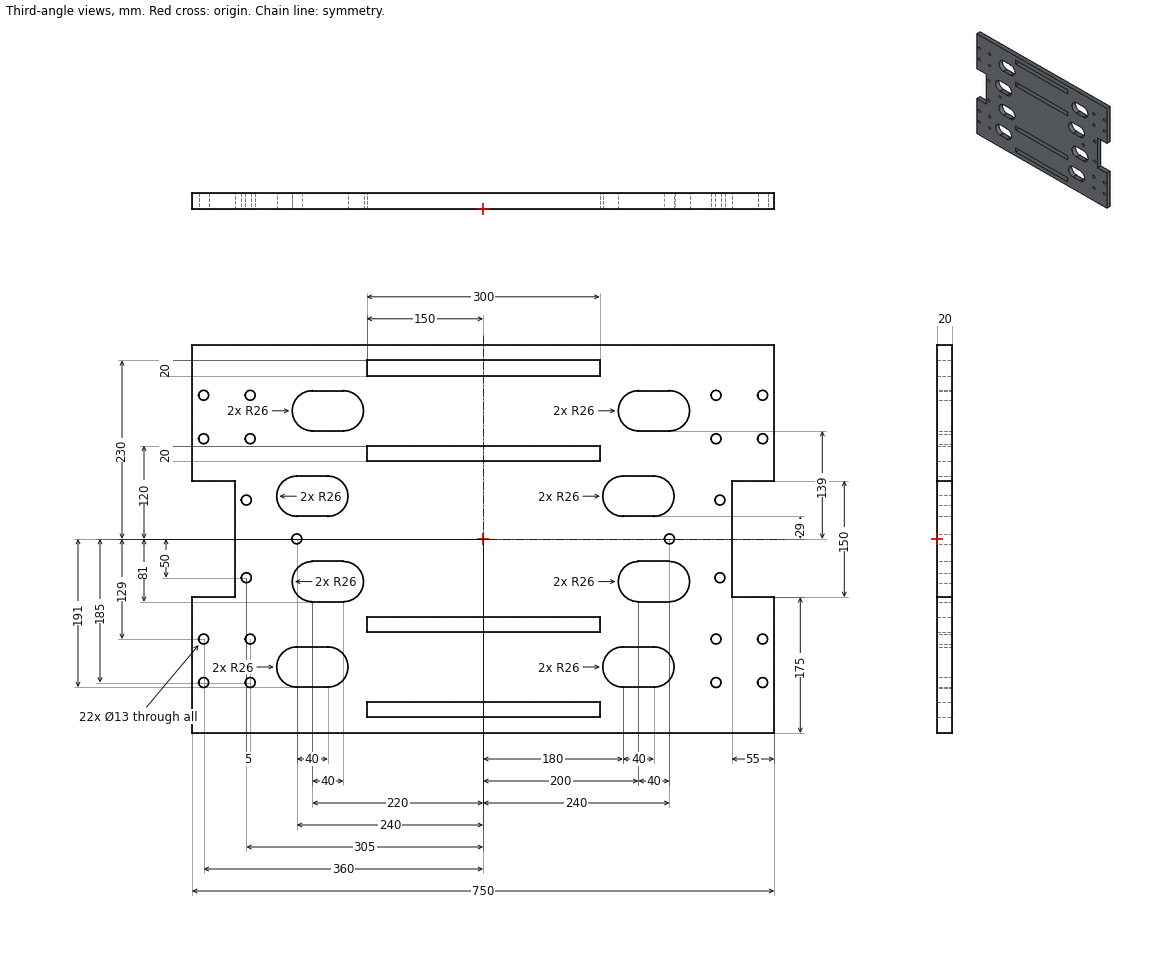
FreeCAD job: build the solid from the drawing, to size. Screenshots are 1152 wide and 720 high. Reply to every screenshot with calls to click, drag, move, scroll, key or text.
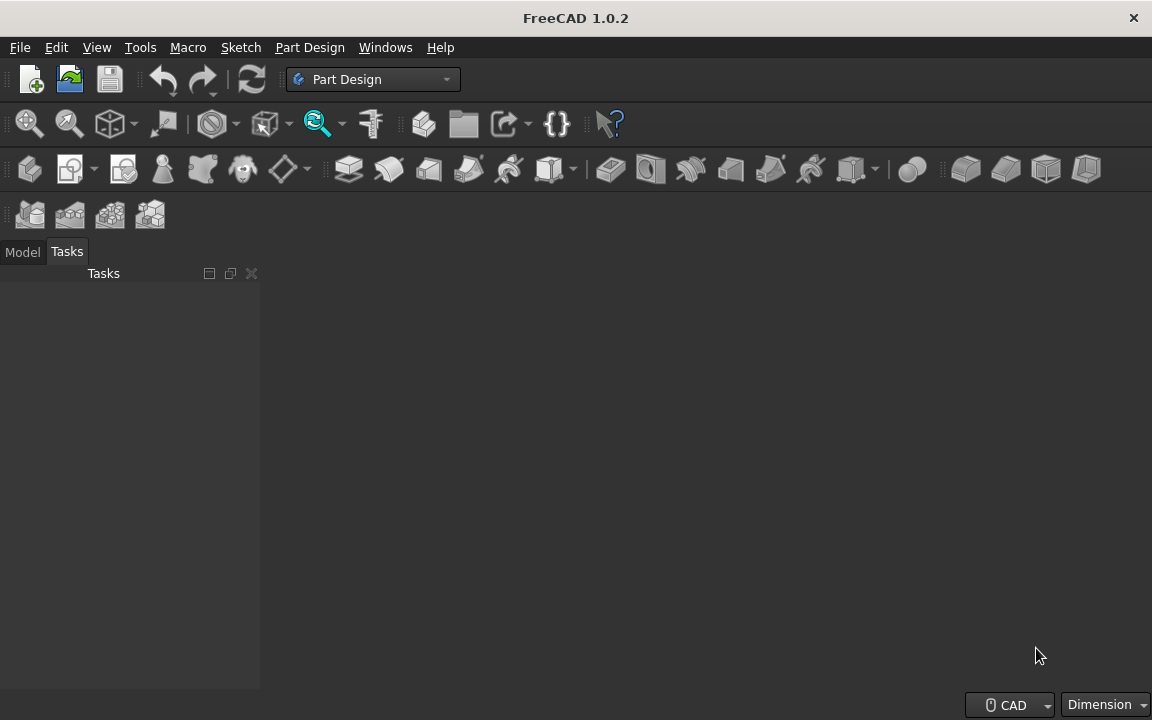
click(30, 80)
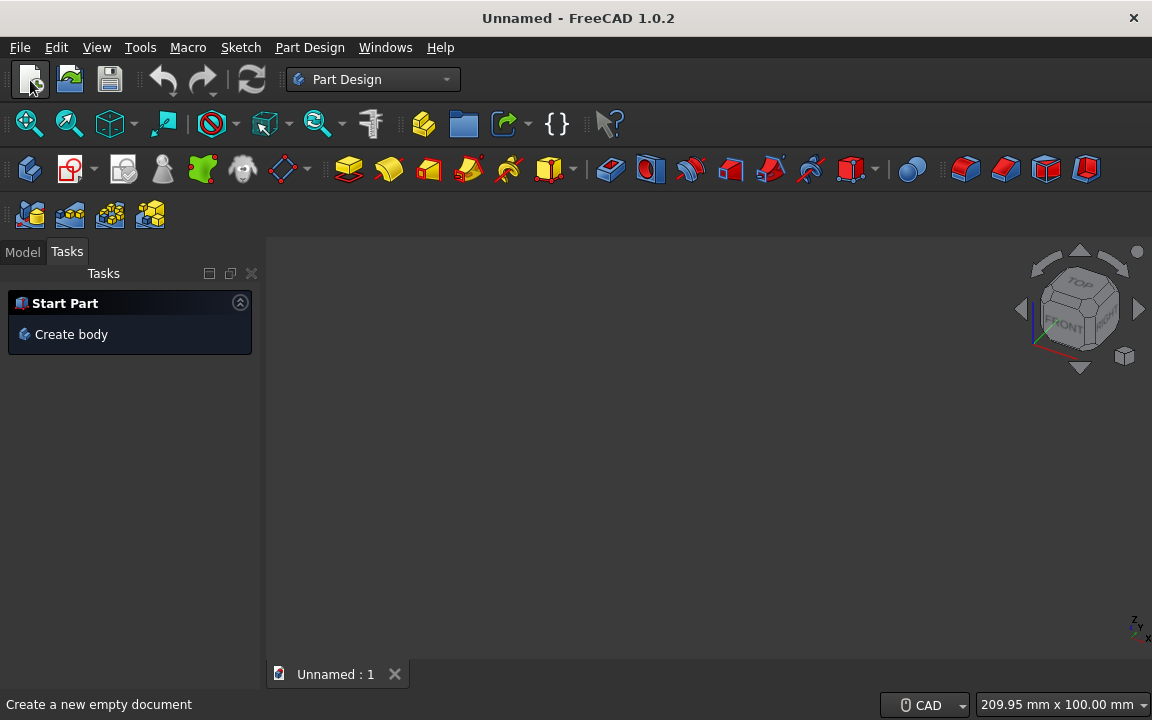
click(70, 170)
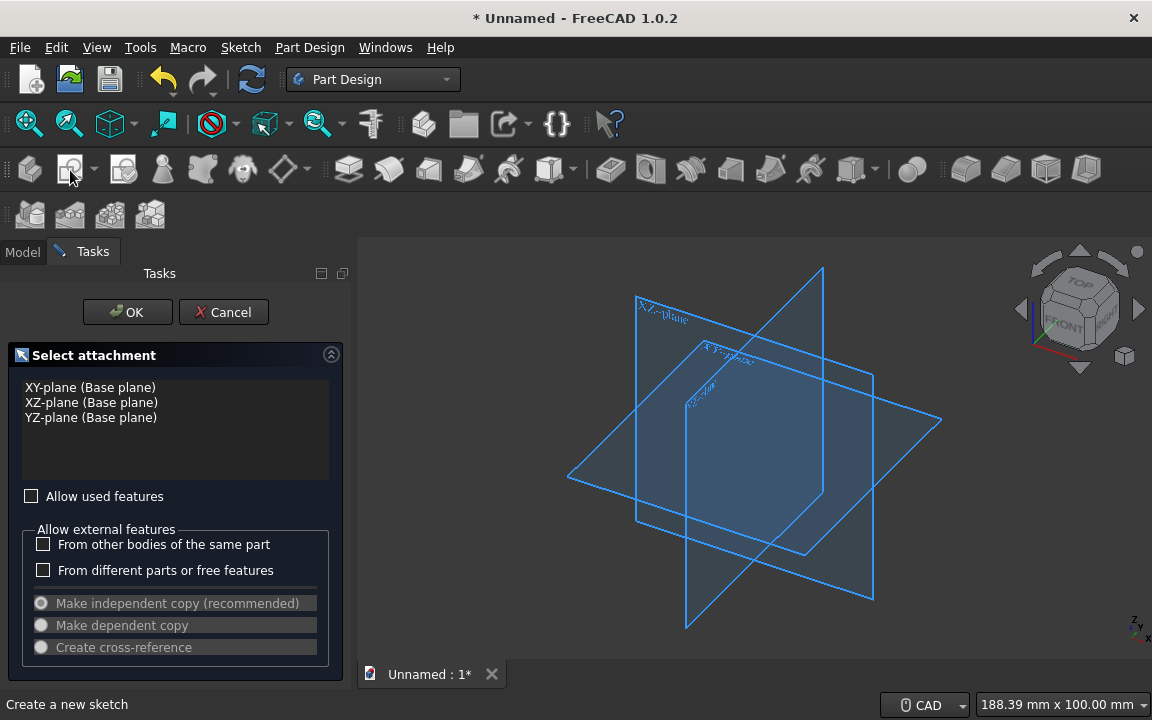
click(82, 402)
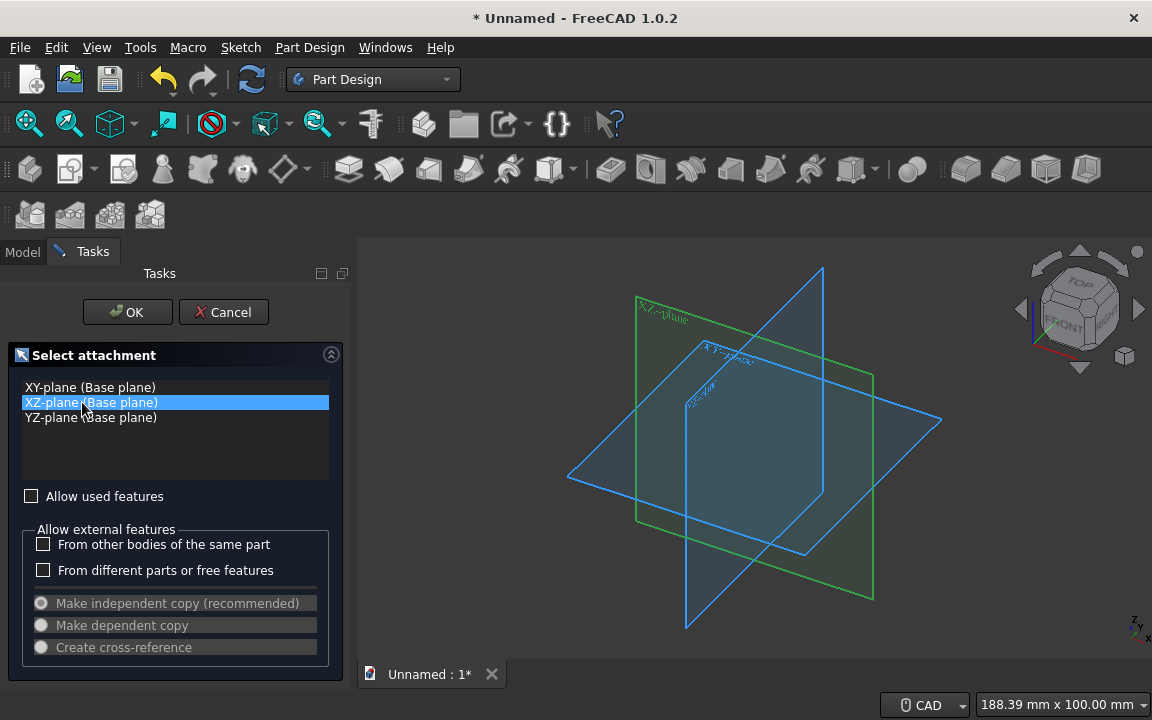
click(128, 312)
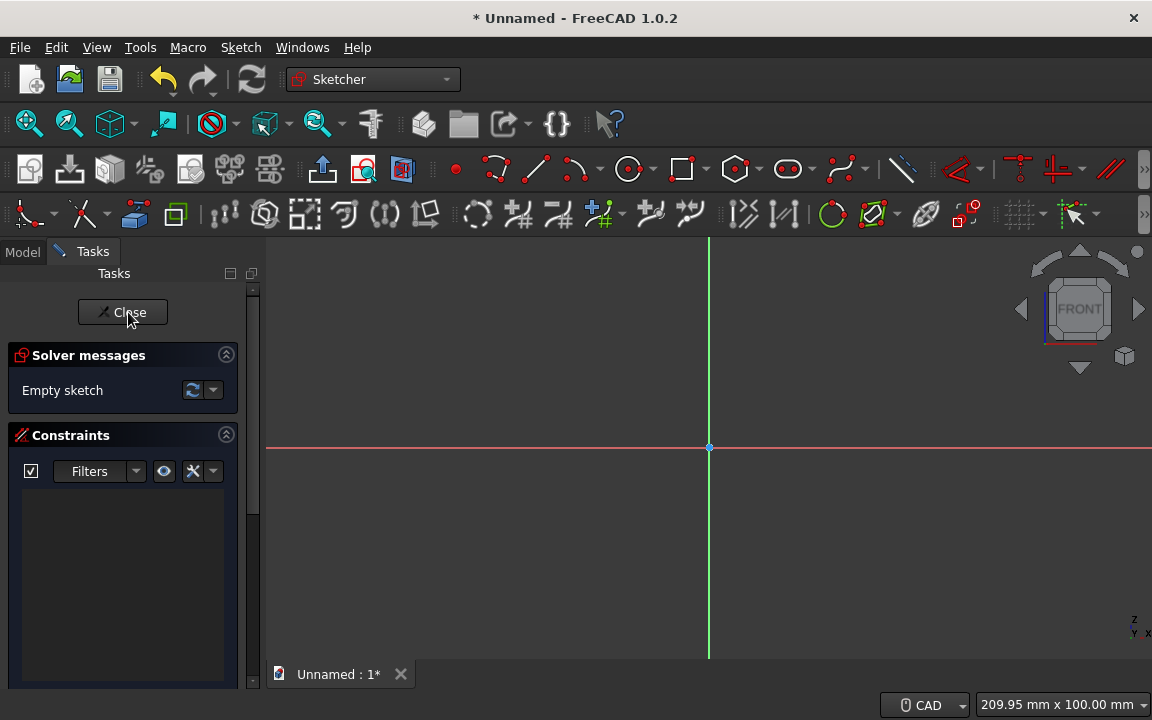
scroll(632, 448, down, 11)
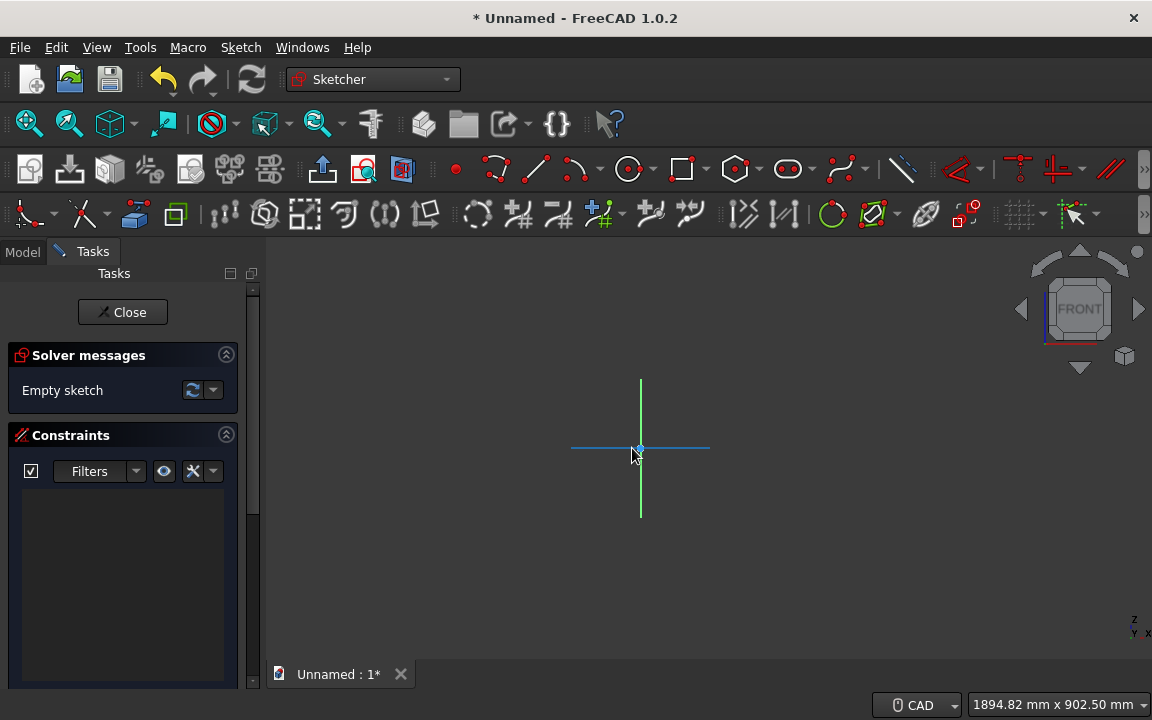
click(496, 170)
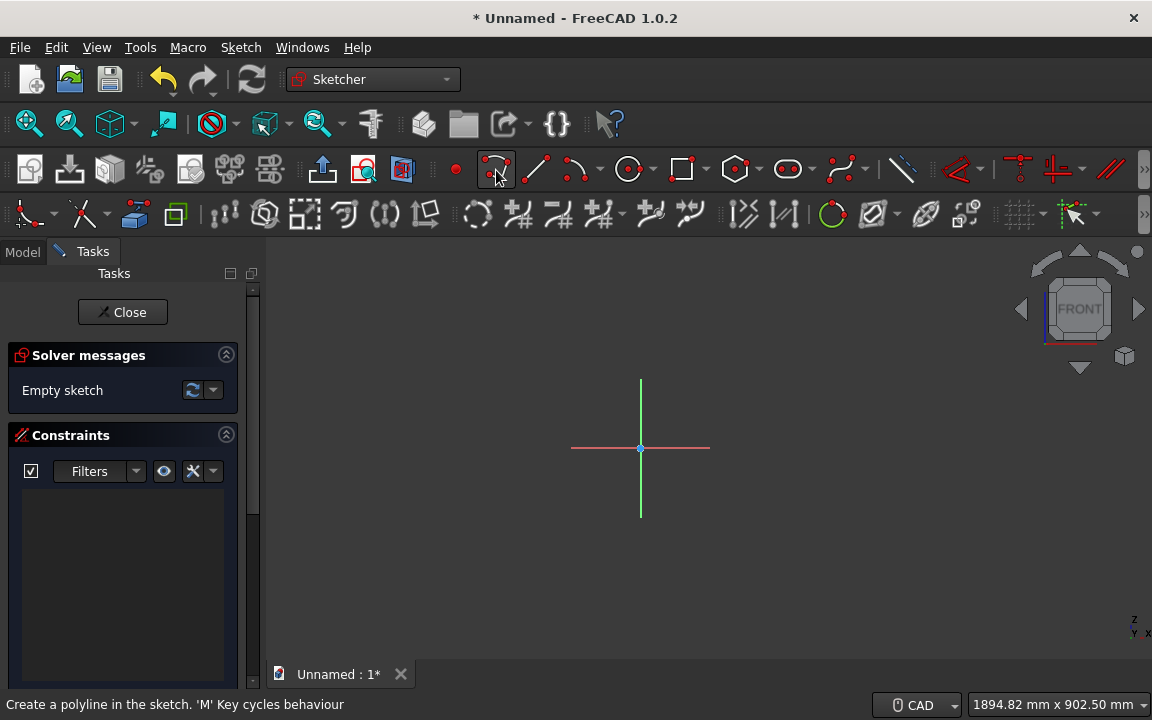
click(791, 413)
click(791, 484)
click(816, 484)
click(816, 565)
click(466, 565)
click(466, 484)
click(491, 484)
click(491, 413)
click(466, 413)
click(466, 332)
click(816, 332)
click(816, 413)
click(791, 414)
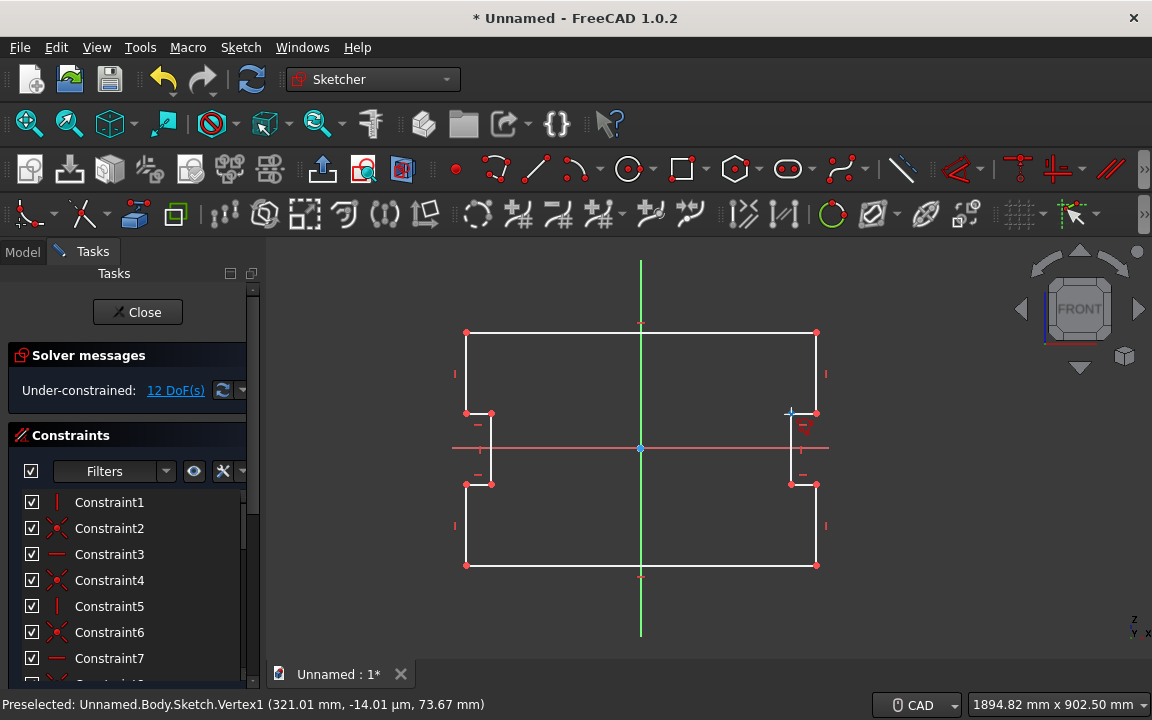
click(682, 170)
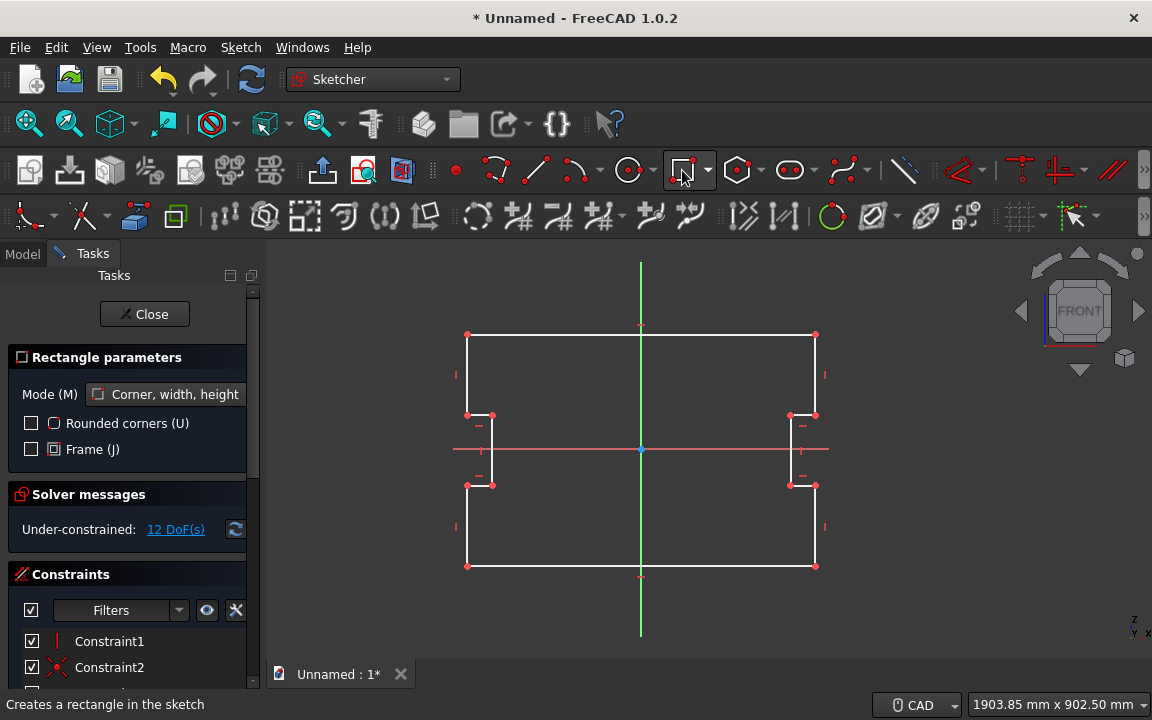
scroll(571, 342, up, 3)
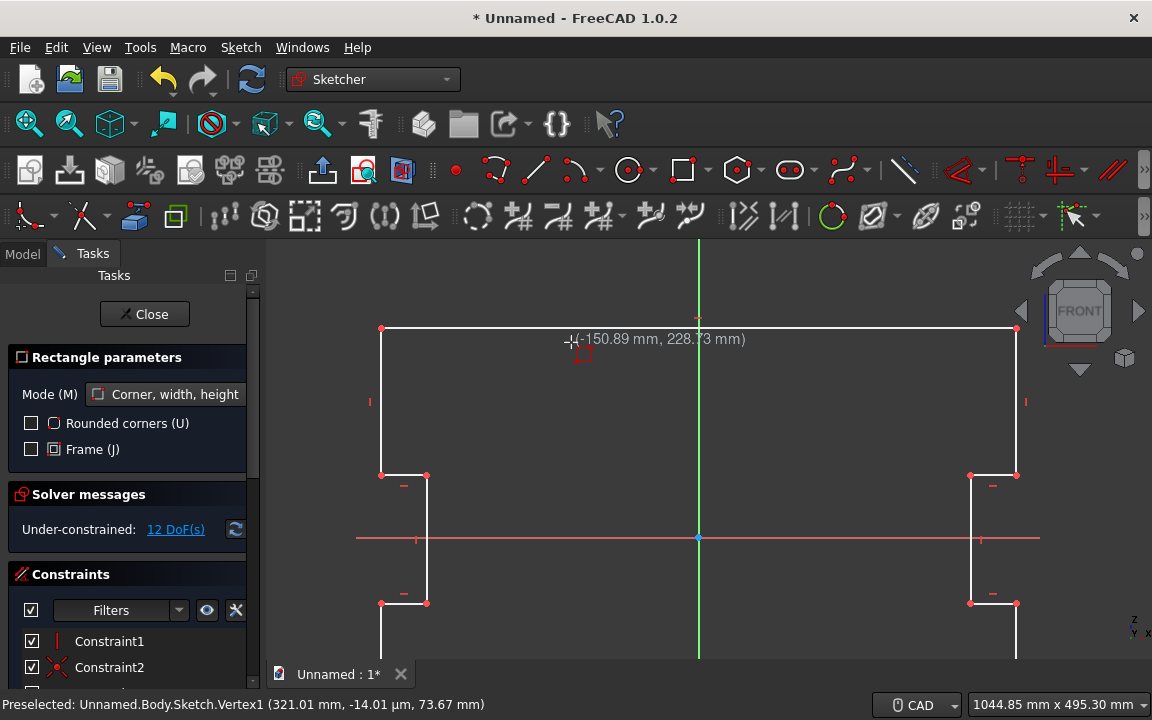
click(571, 343)
click(826, 360)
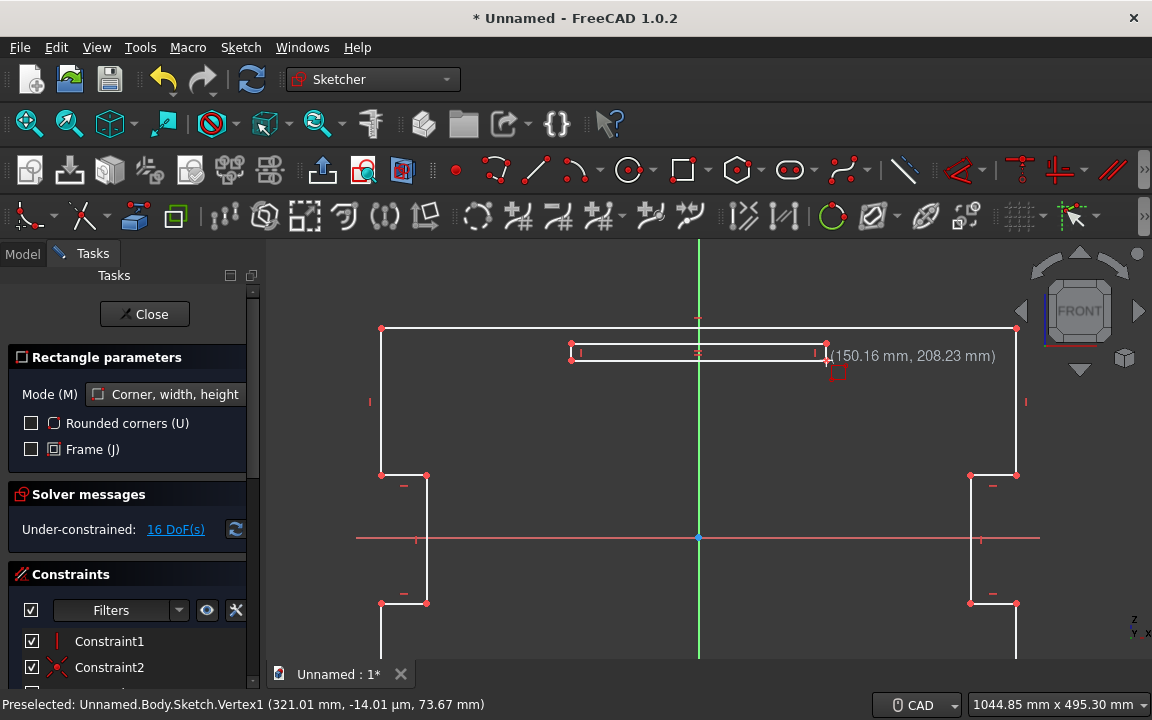
click(571, 436)
click(826, 453)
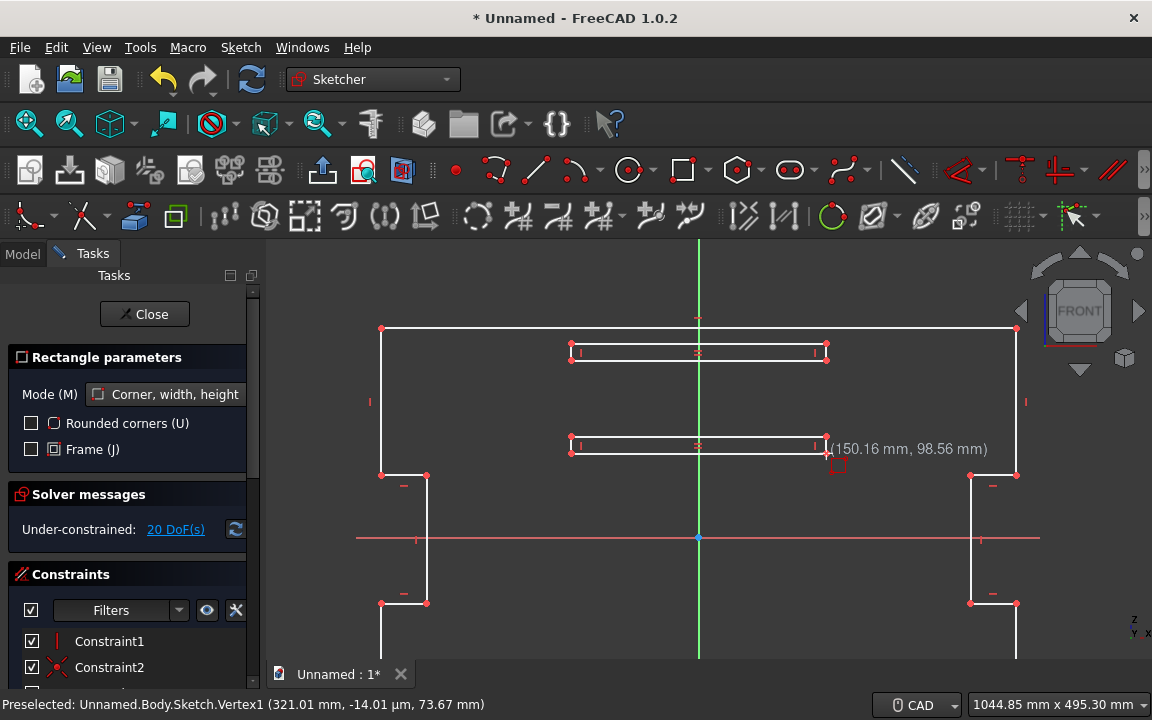
click(571, 622)